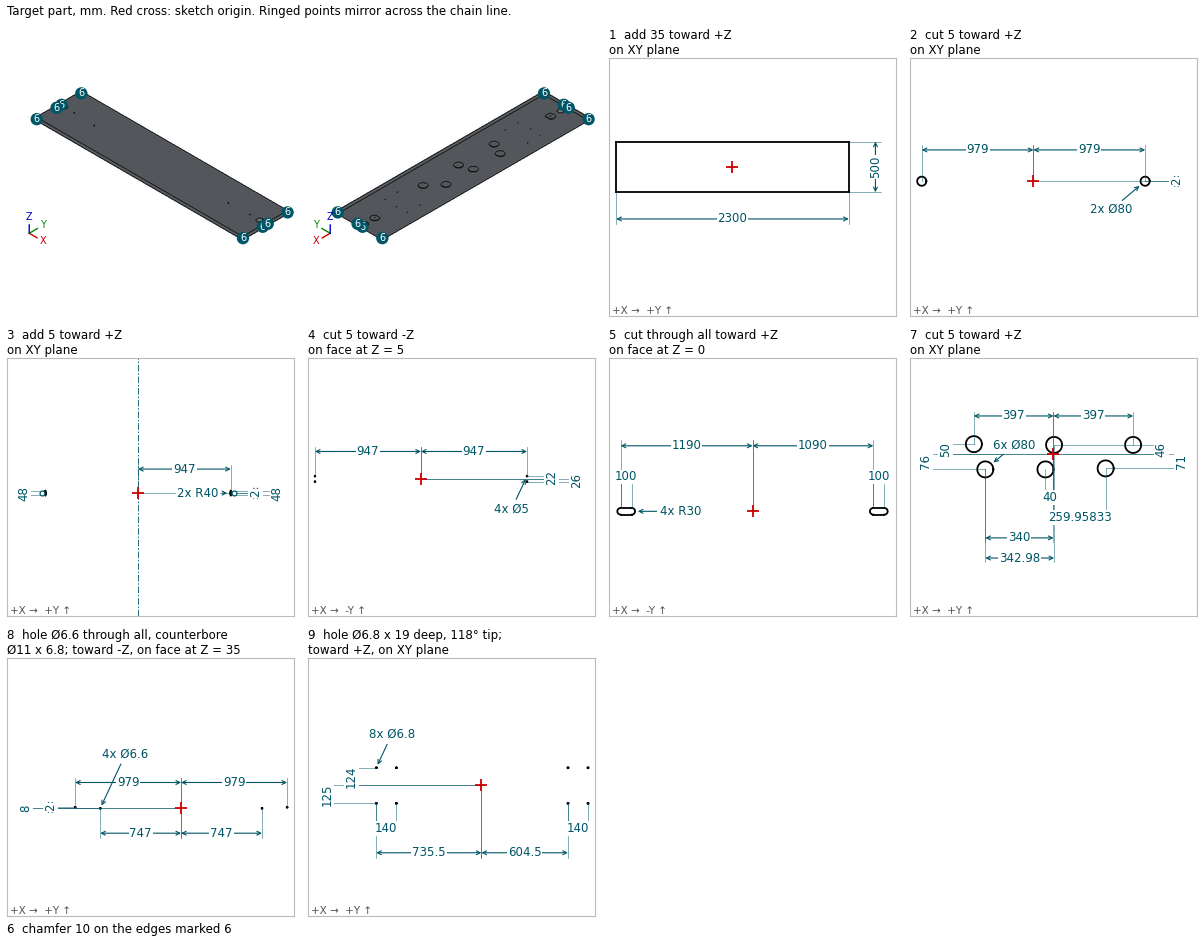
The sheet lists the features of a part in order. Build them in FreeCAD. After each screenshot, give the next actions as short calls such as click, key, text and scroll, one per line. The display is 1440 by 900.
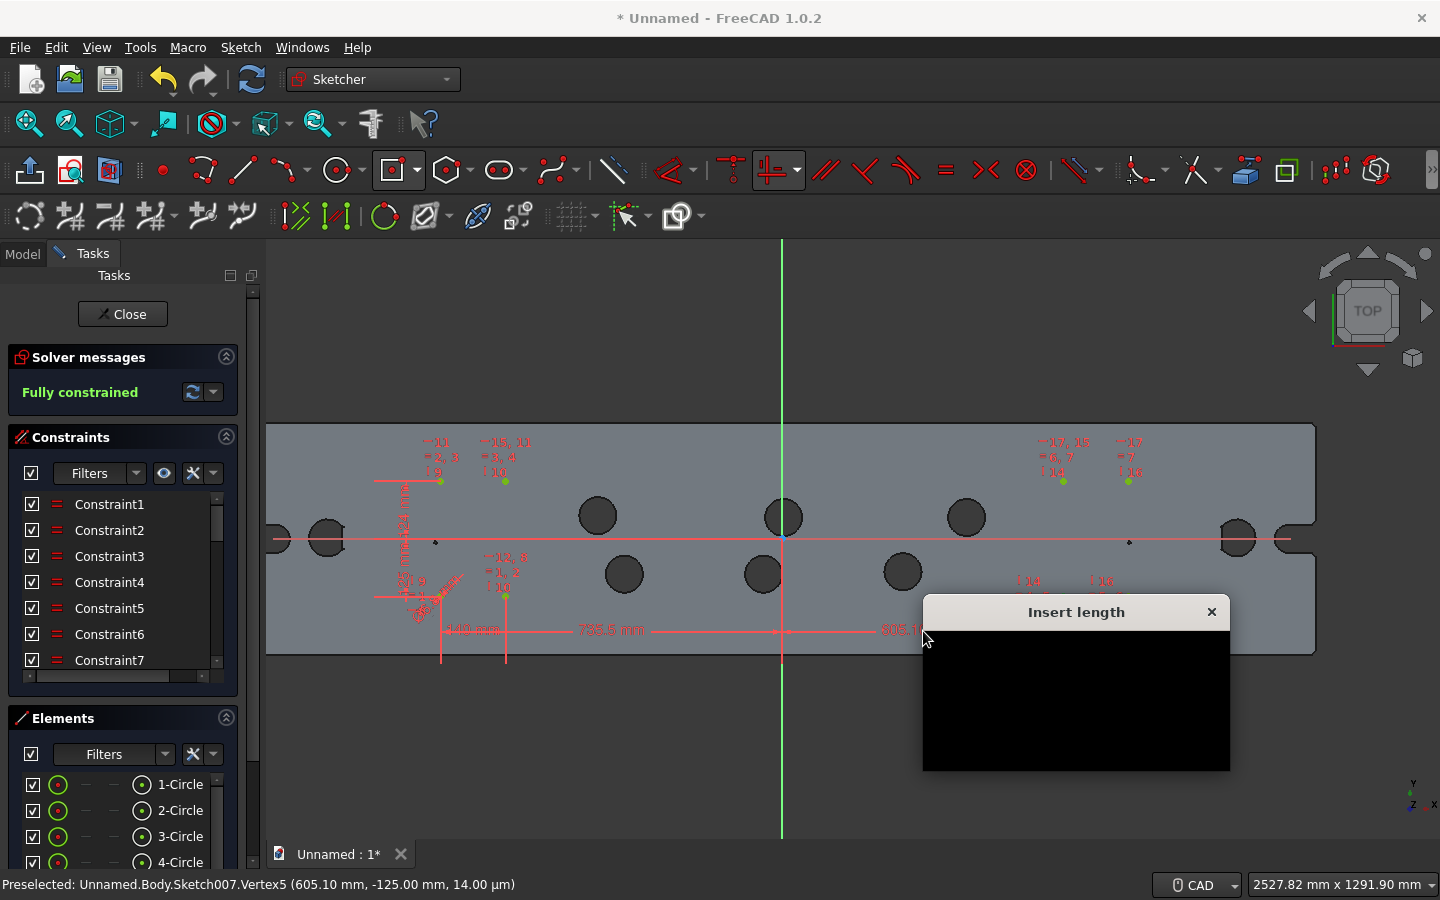
text(604.5)
key(Return)
key(Escape)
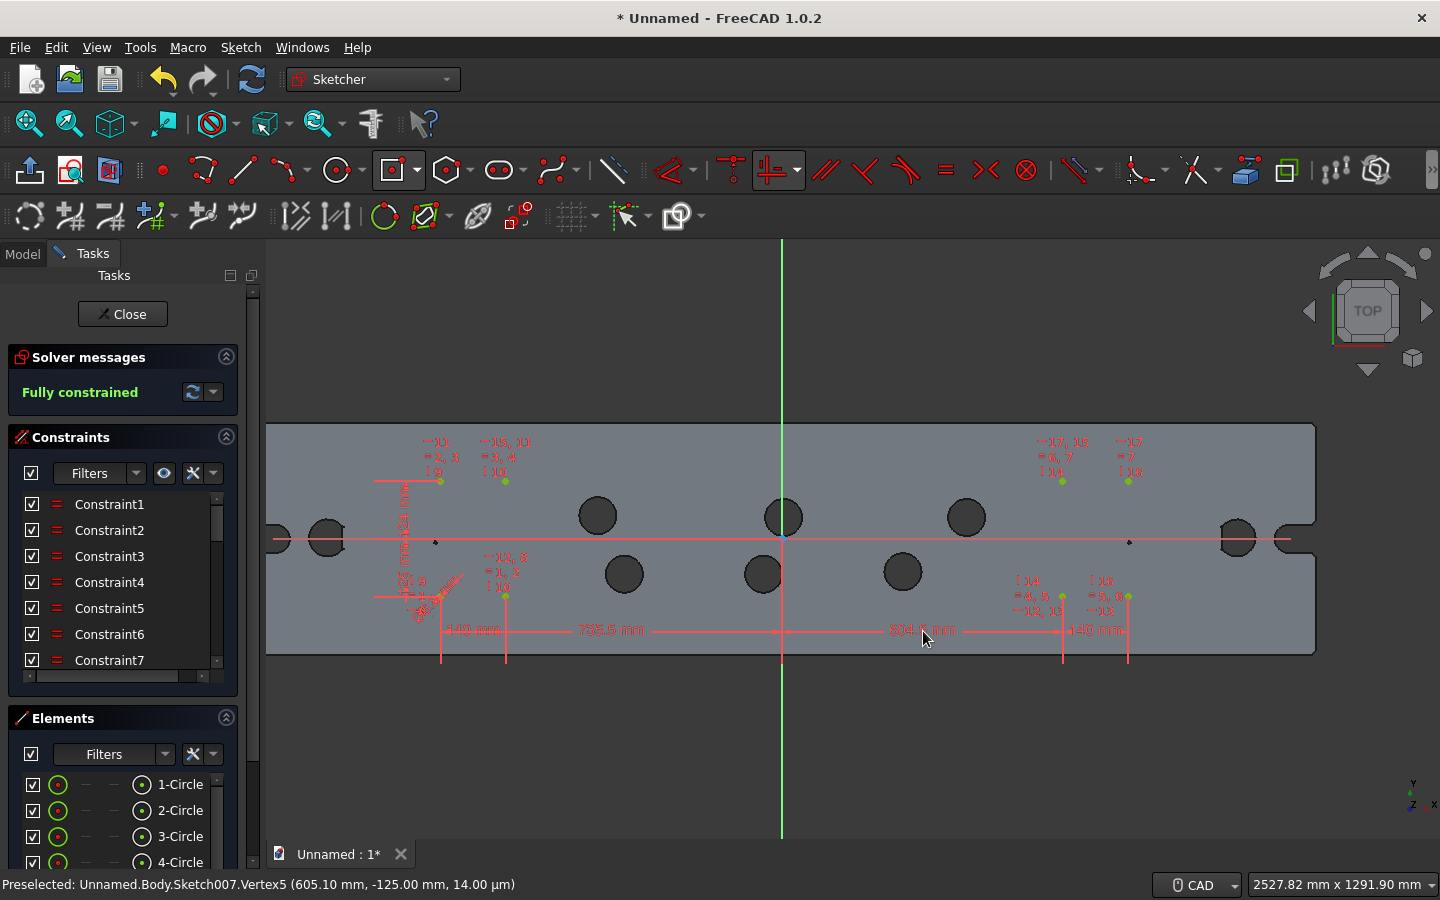
click(123, 314)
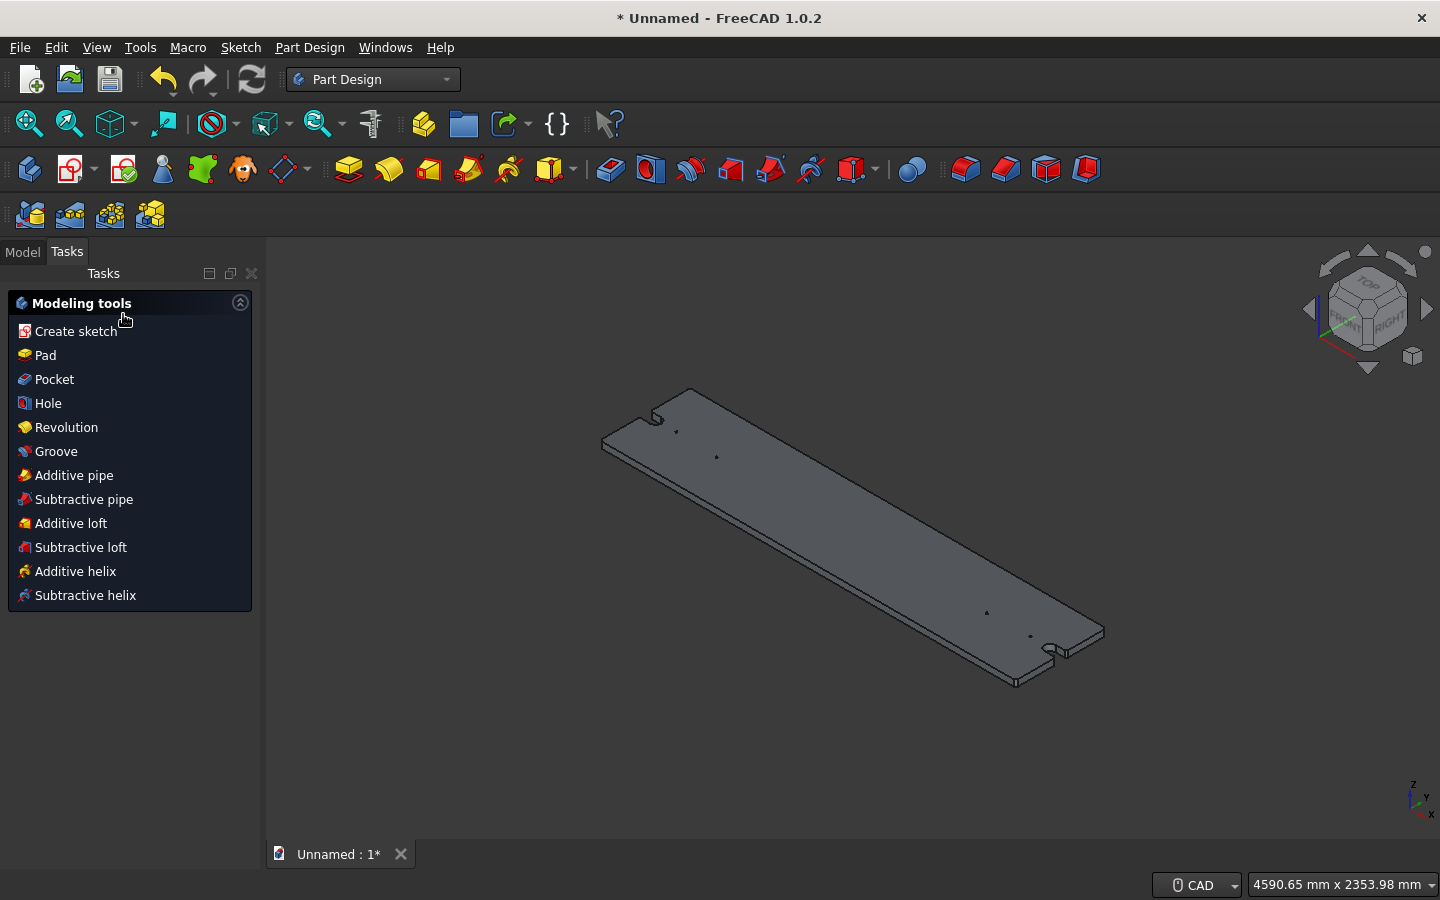
click(652, 170)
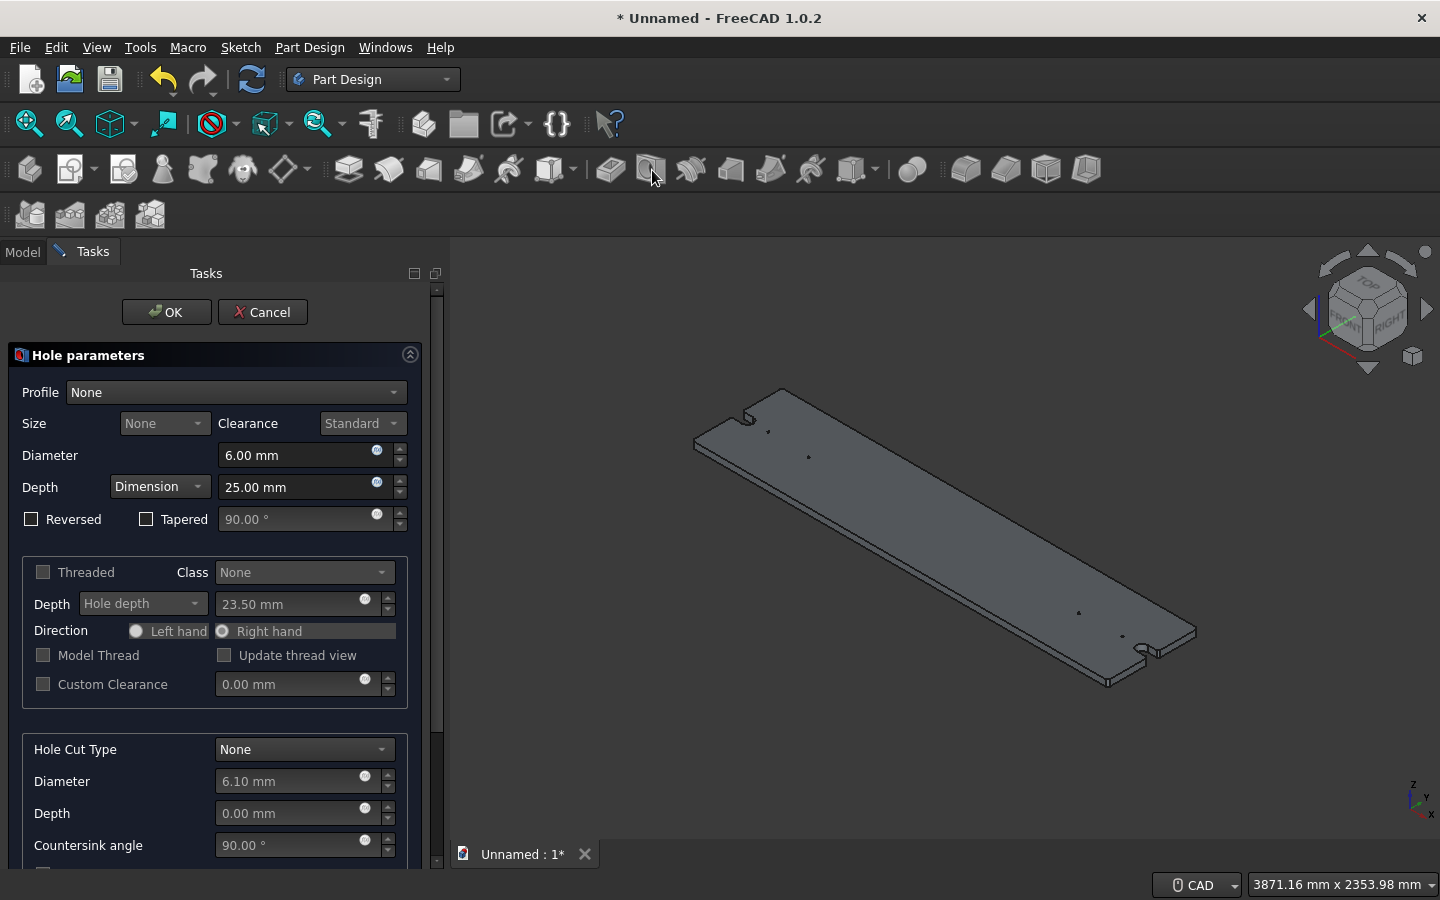
triple_click(305, 455)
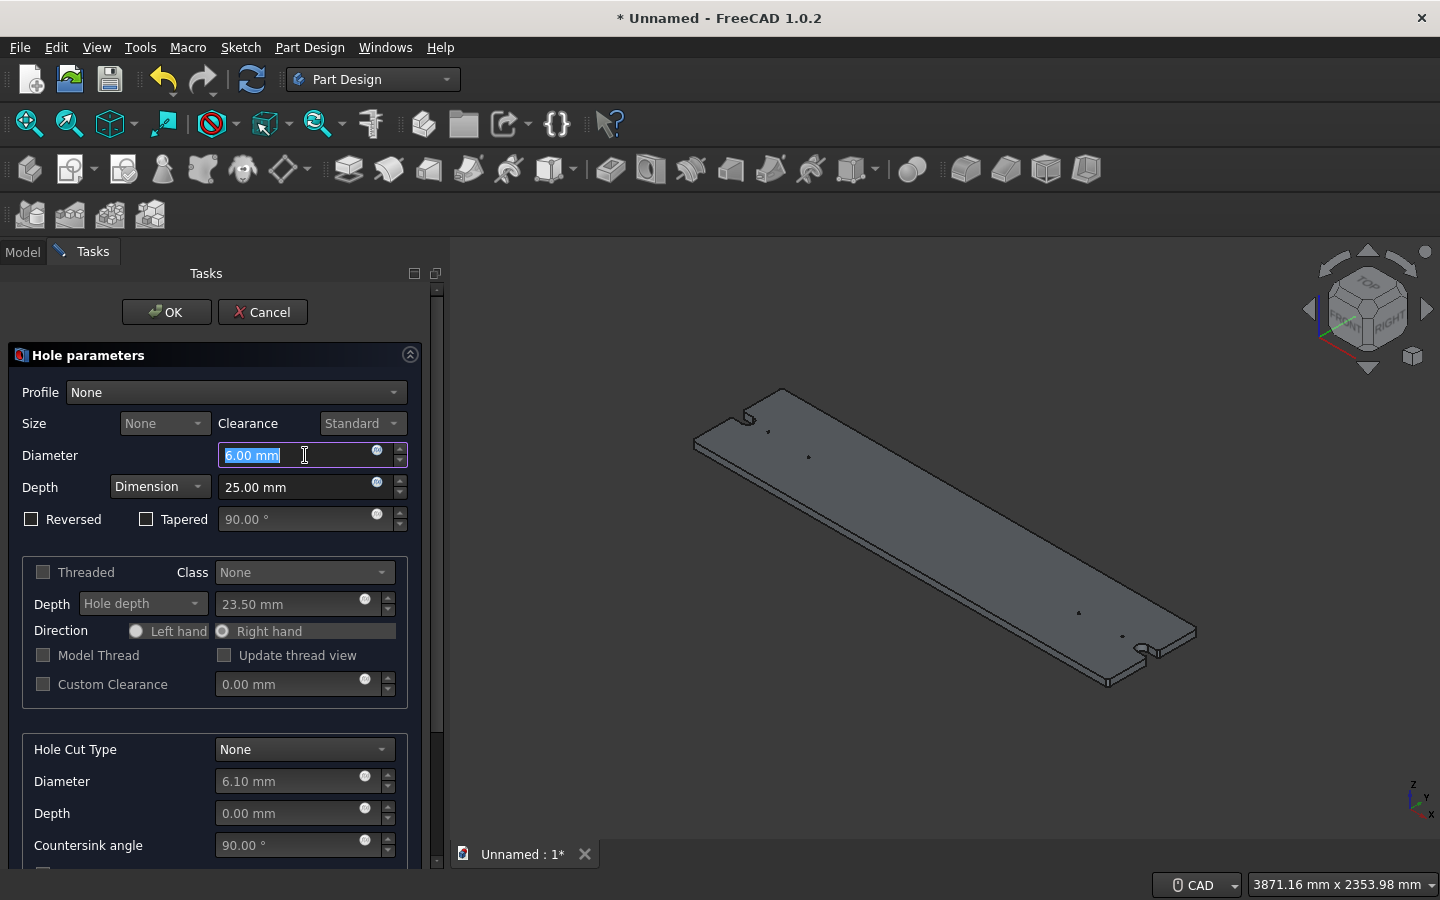
text(6.8)
key(Tab)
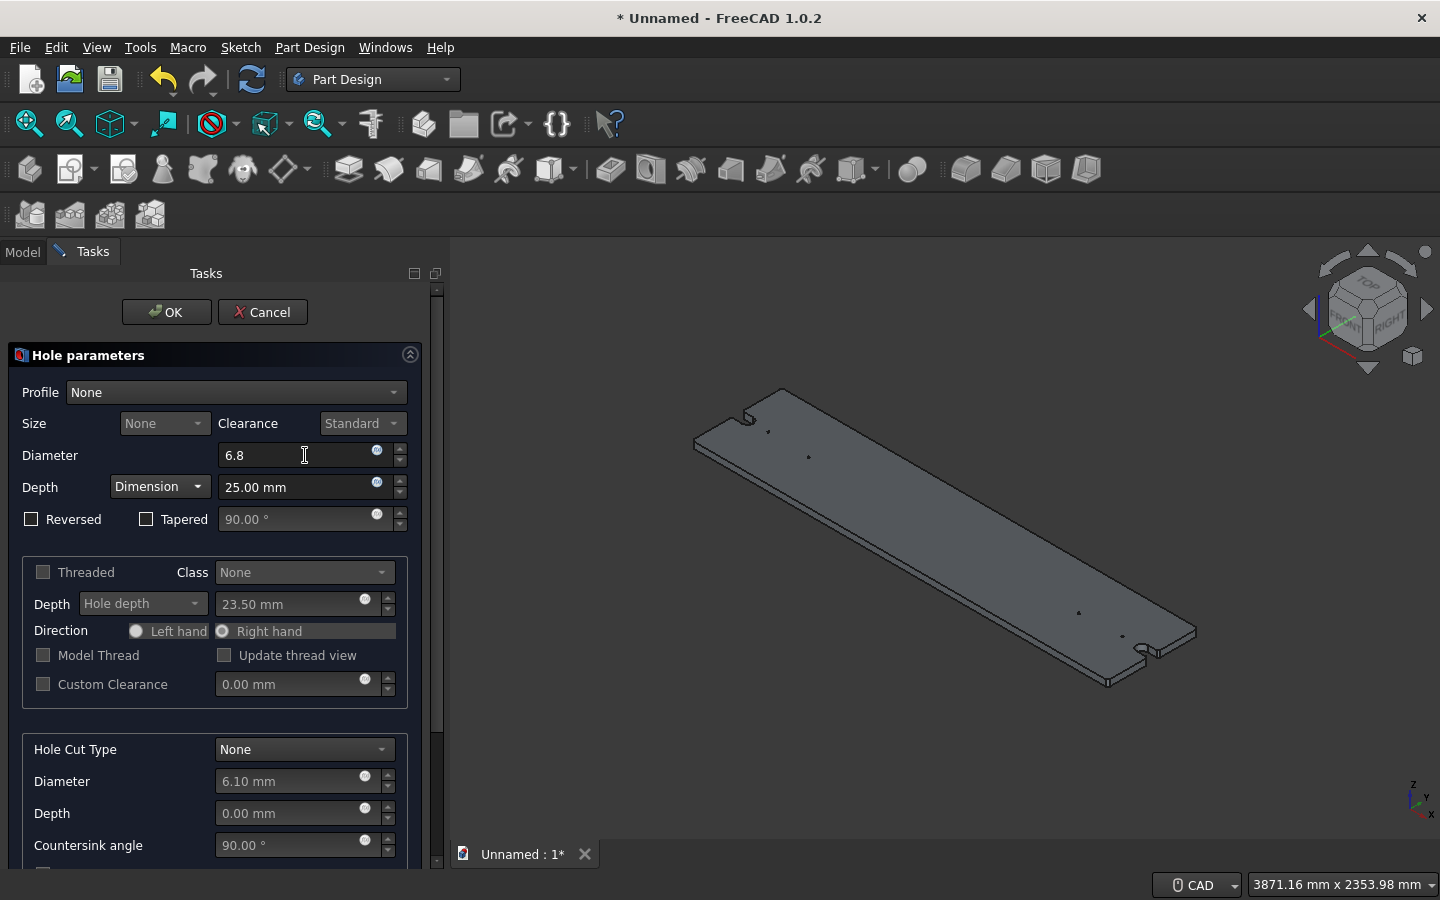
triple_click(305, 487)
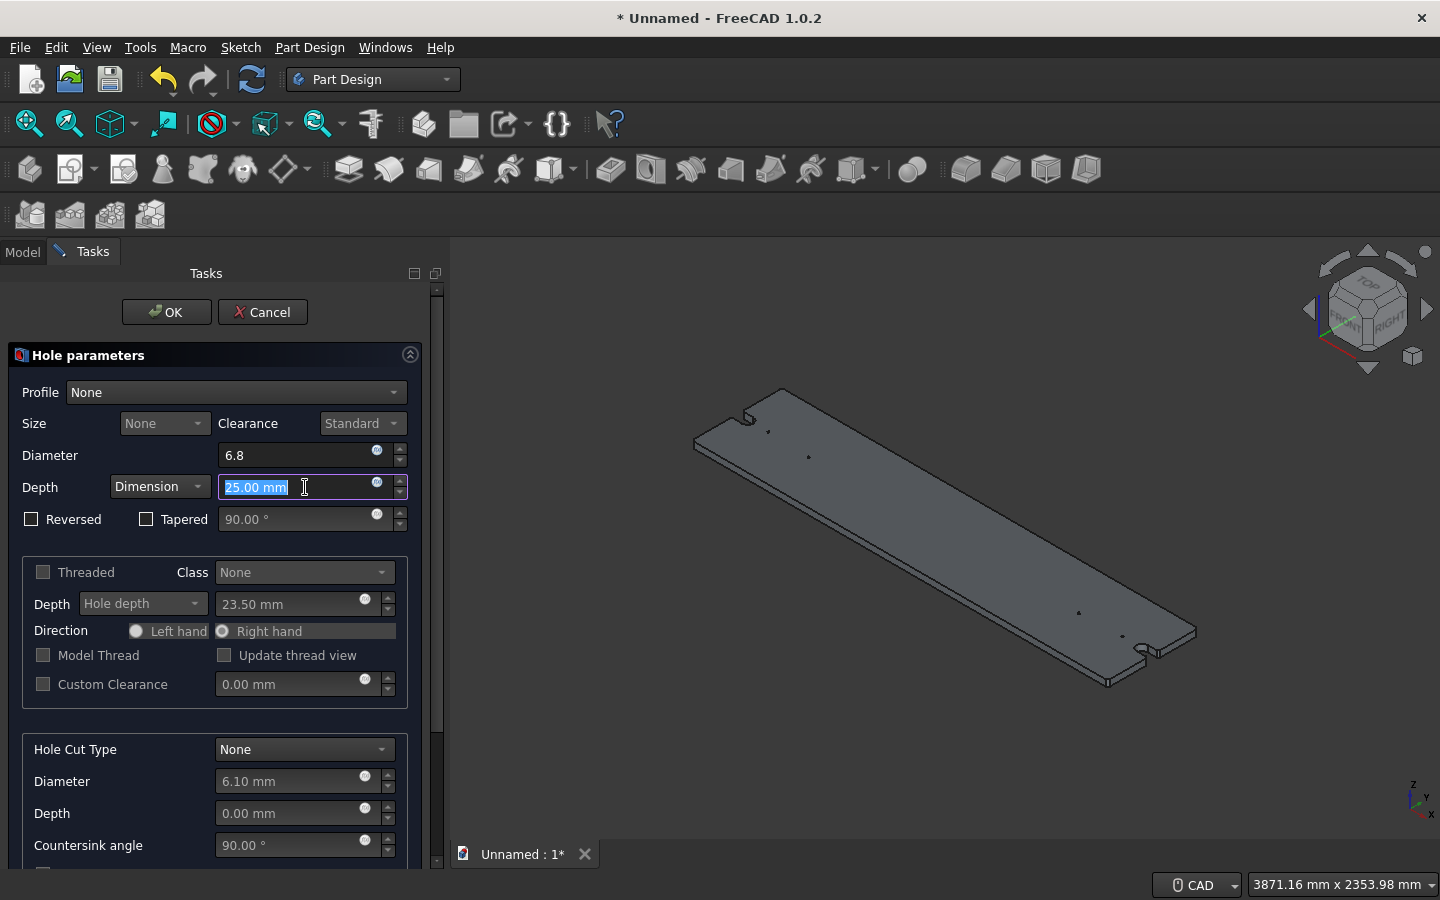
text(19)
key(Tab)